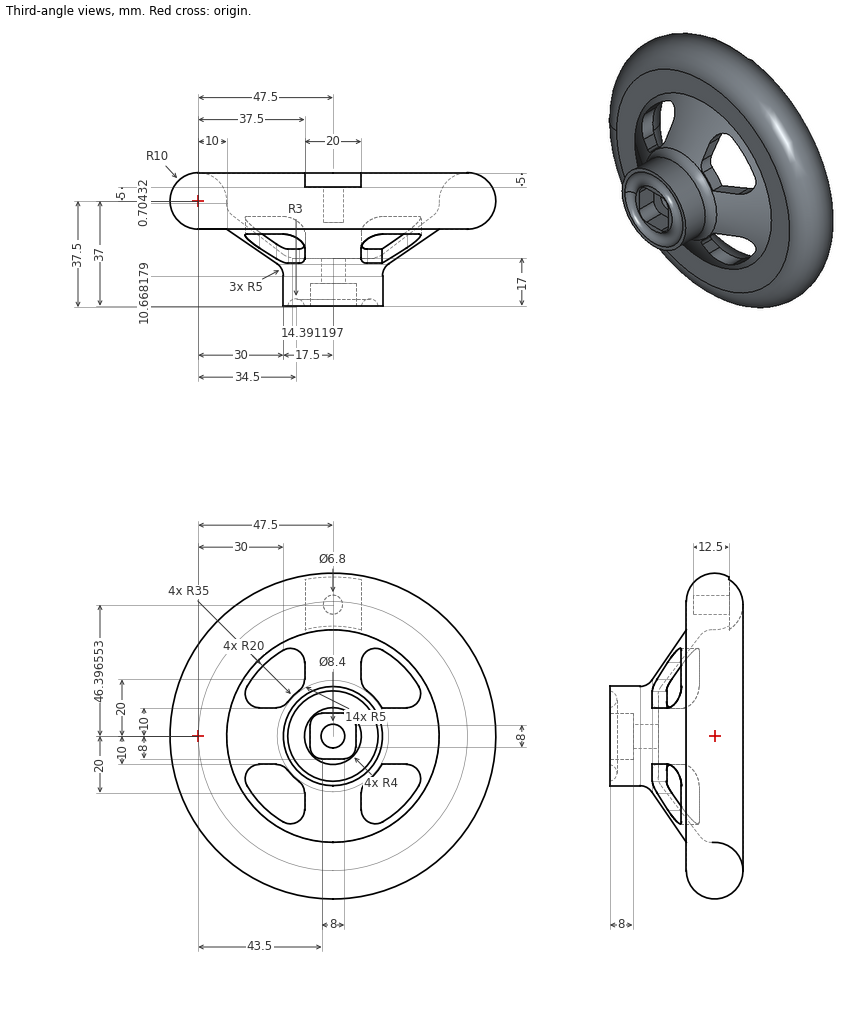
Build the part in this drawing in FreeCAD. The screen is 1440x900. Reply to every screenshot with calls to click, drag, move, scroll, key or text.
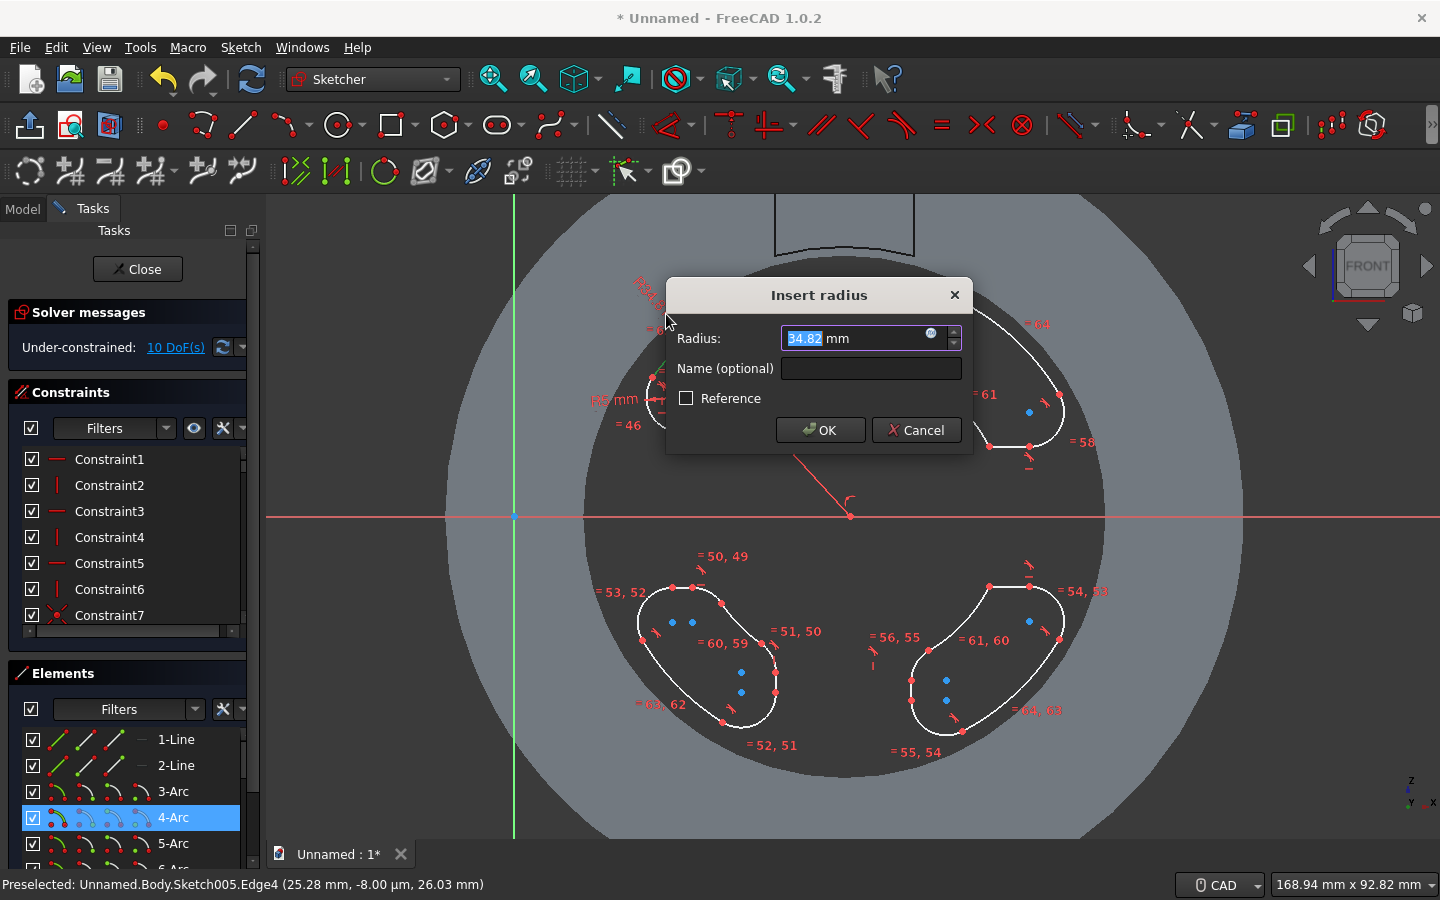
text(35)
key(Return)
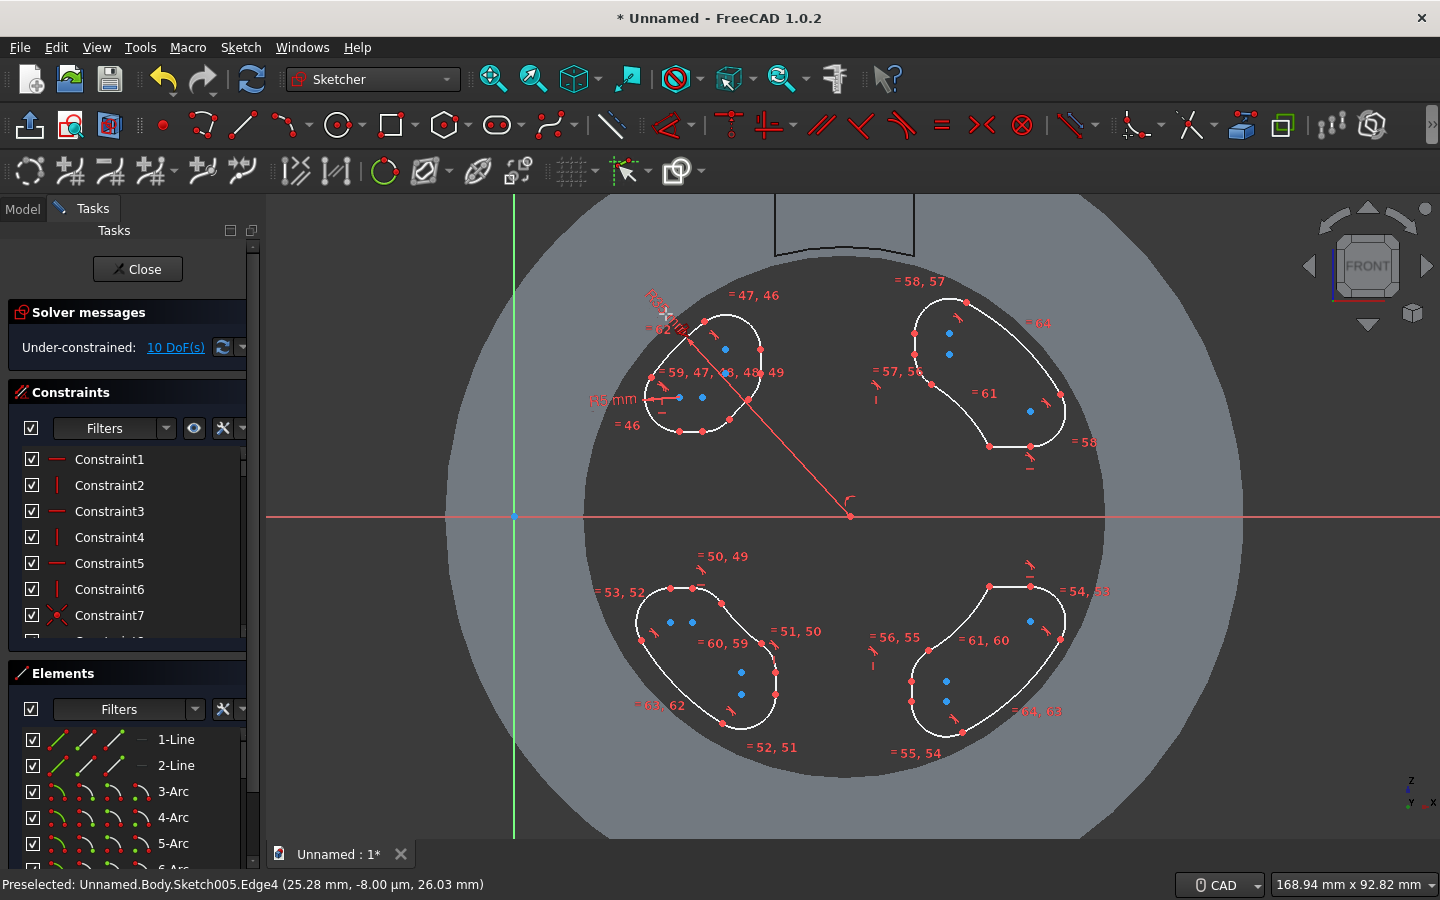
click(739, 409)
click(716, 387)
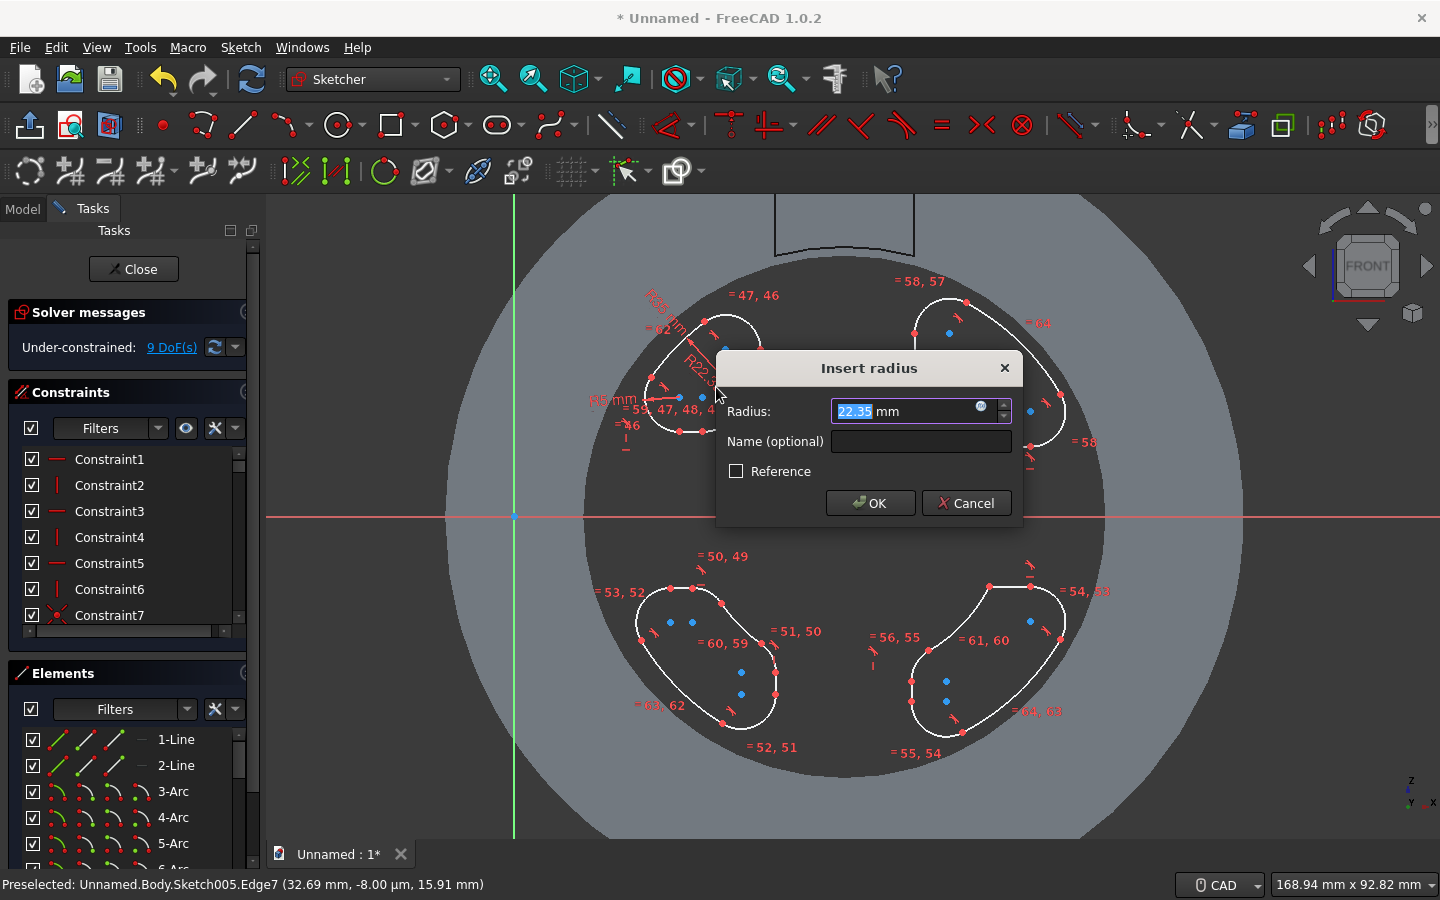
text(20)
key(Return)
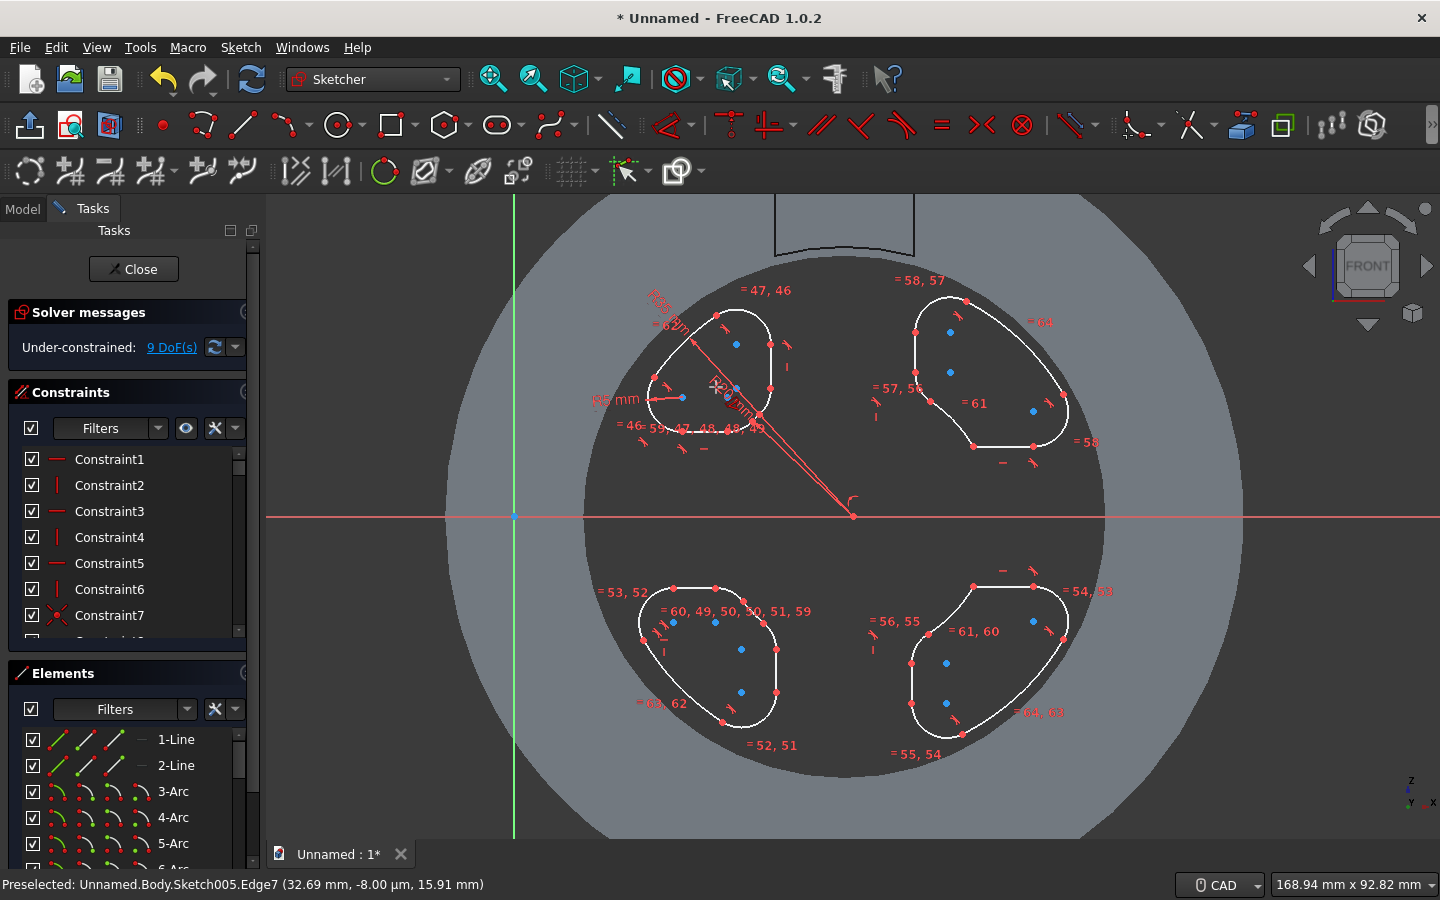
click(727, 432)
click(480, 474)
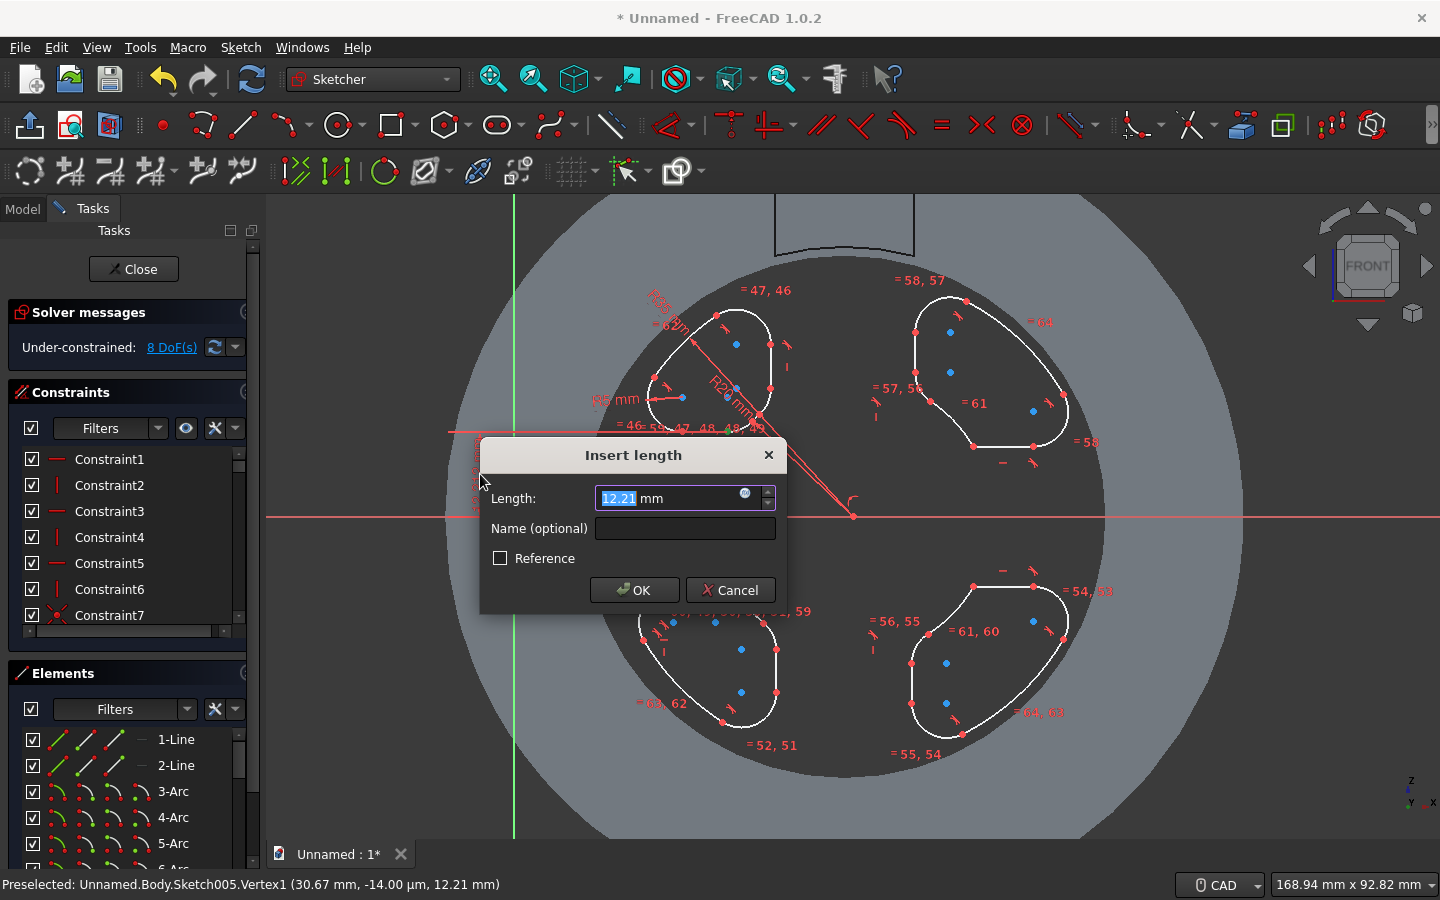
text(10)
key(Return)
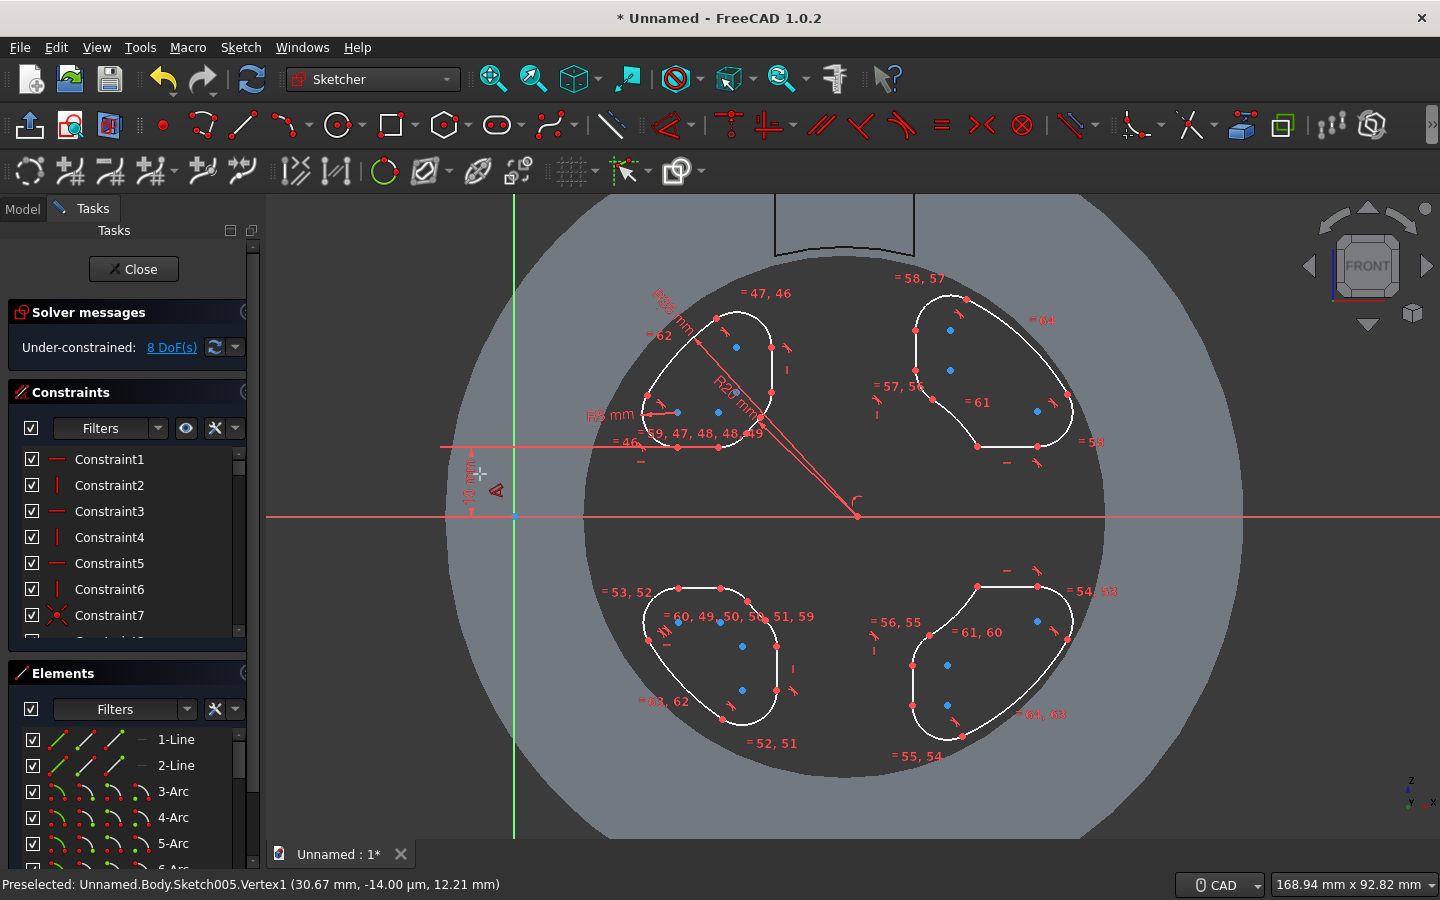
click(772, 392)
click(480, 426)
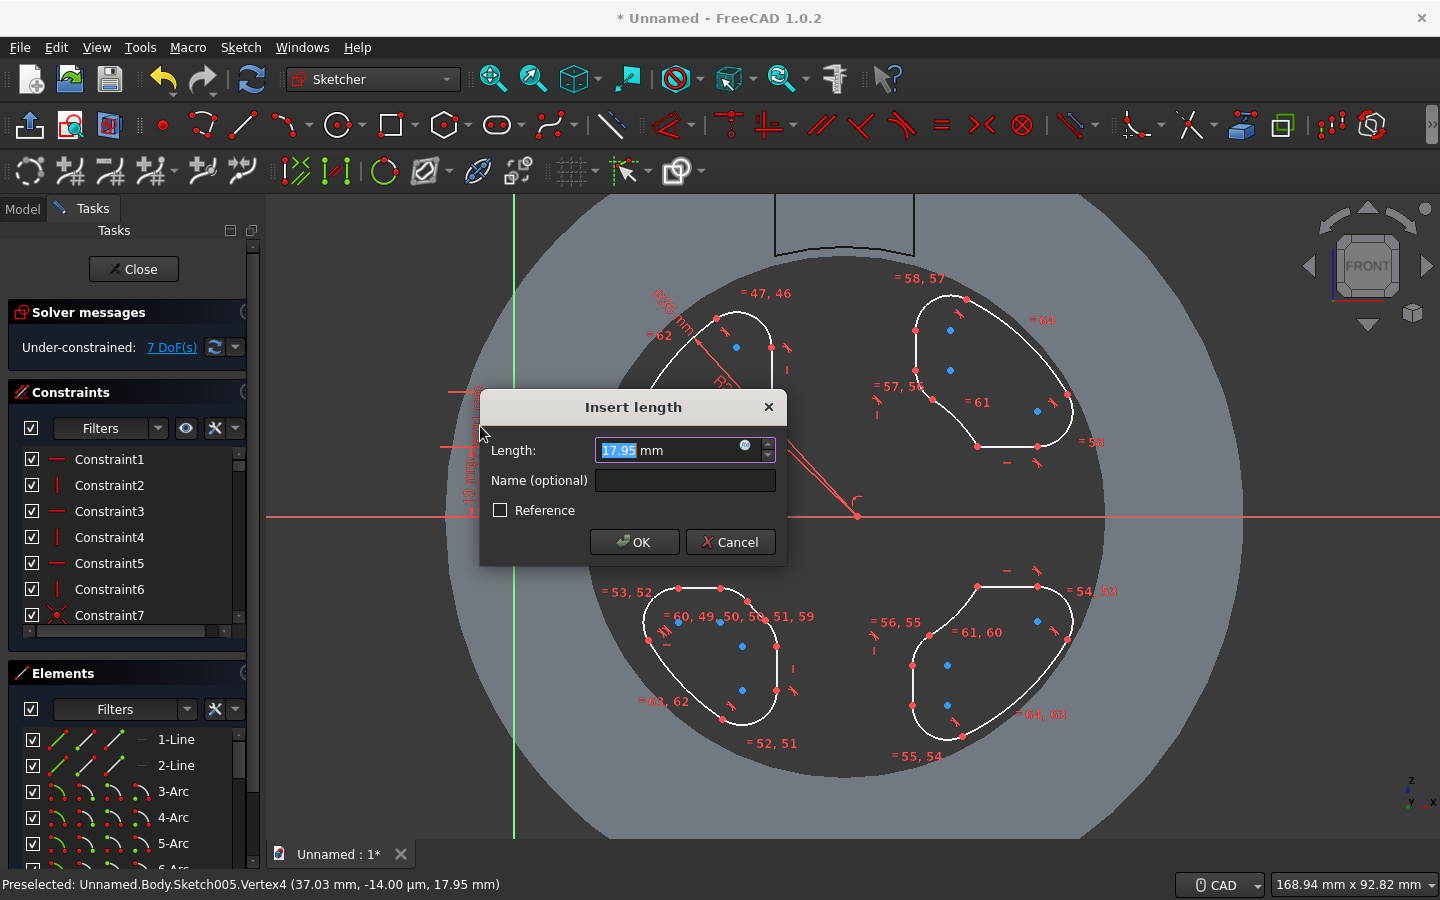
text(20)
key(Return)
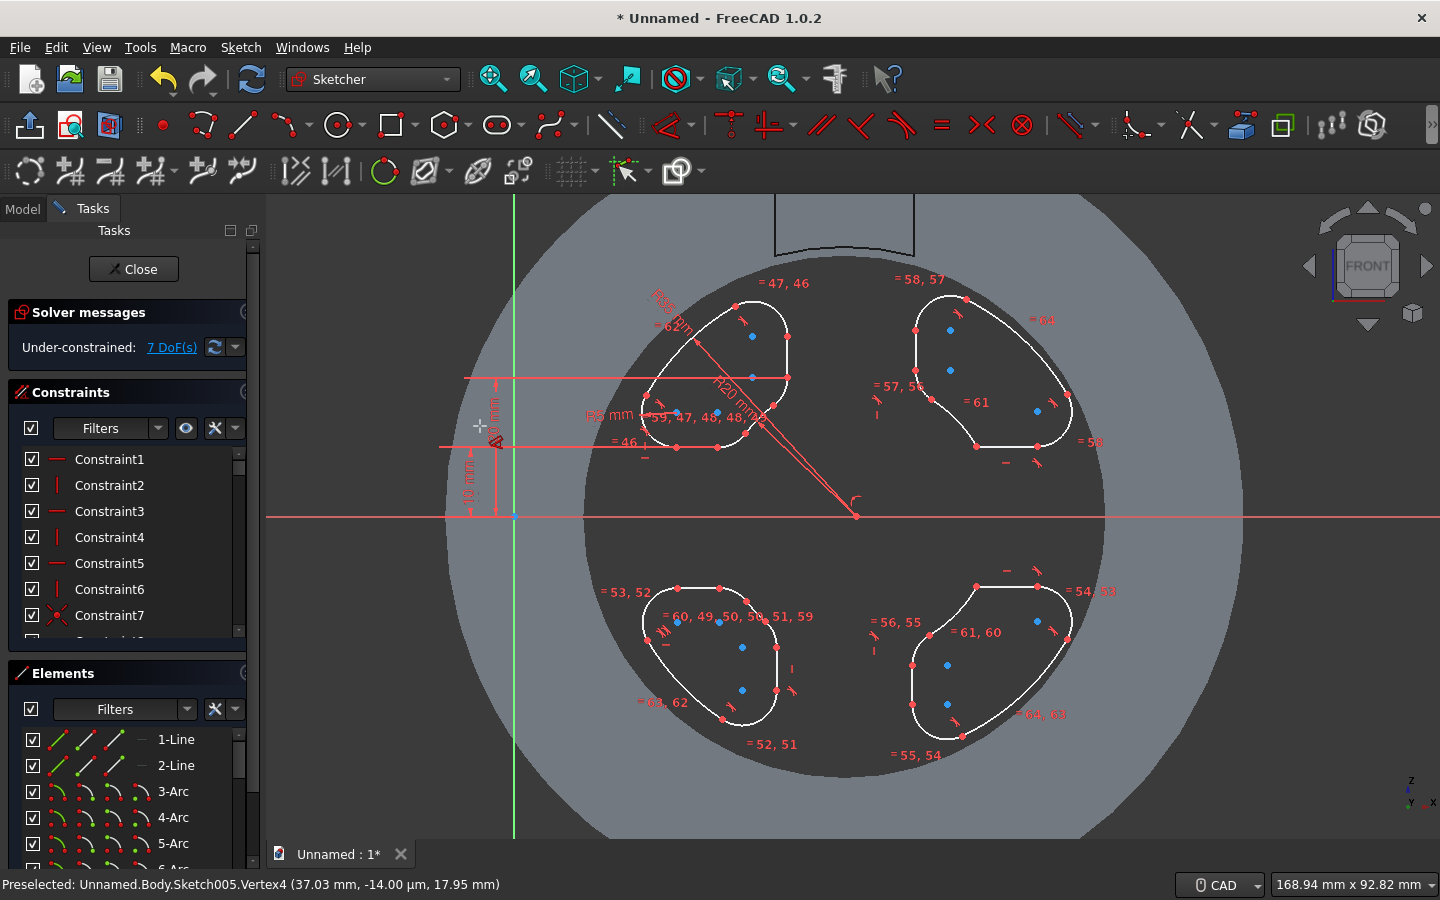
click(735, 306)
click(625, 272)